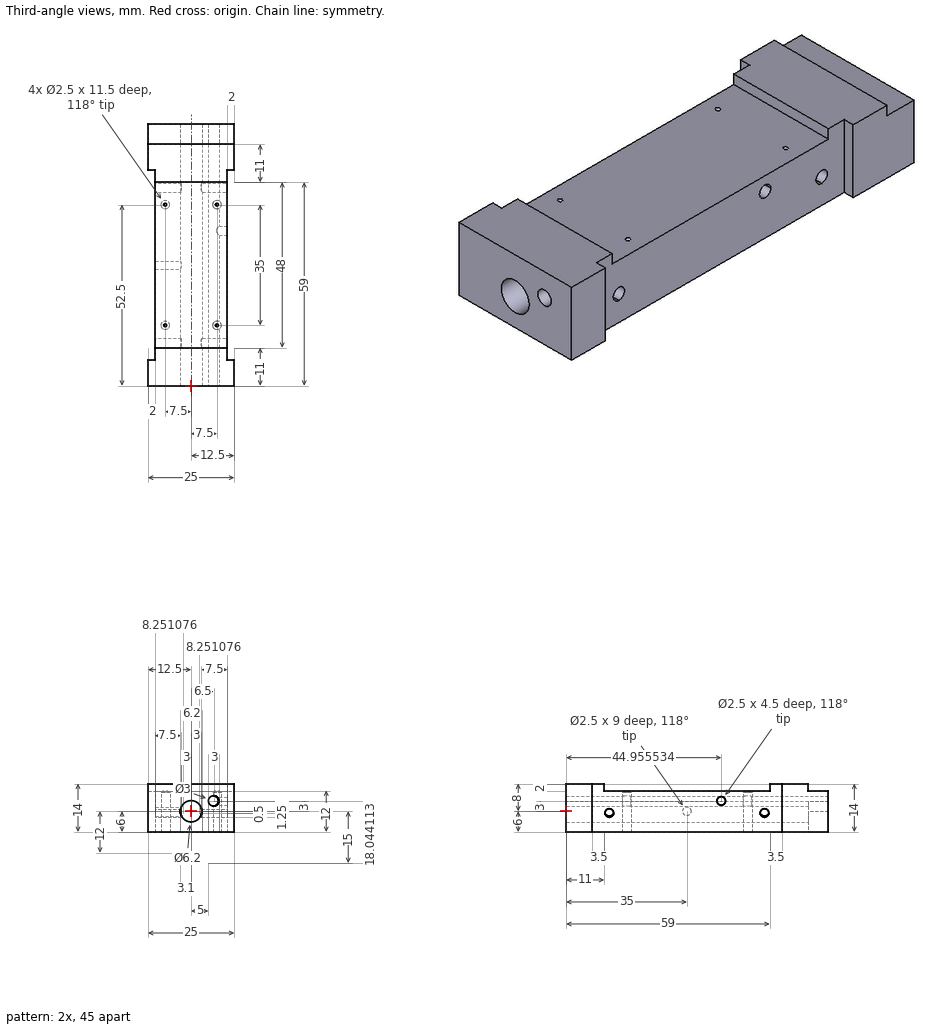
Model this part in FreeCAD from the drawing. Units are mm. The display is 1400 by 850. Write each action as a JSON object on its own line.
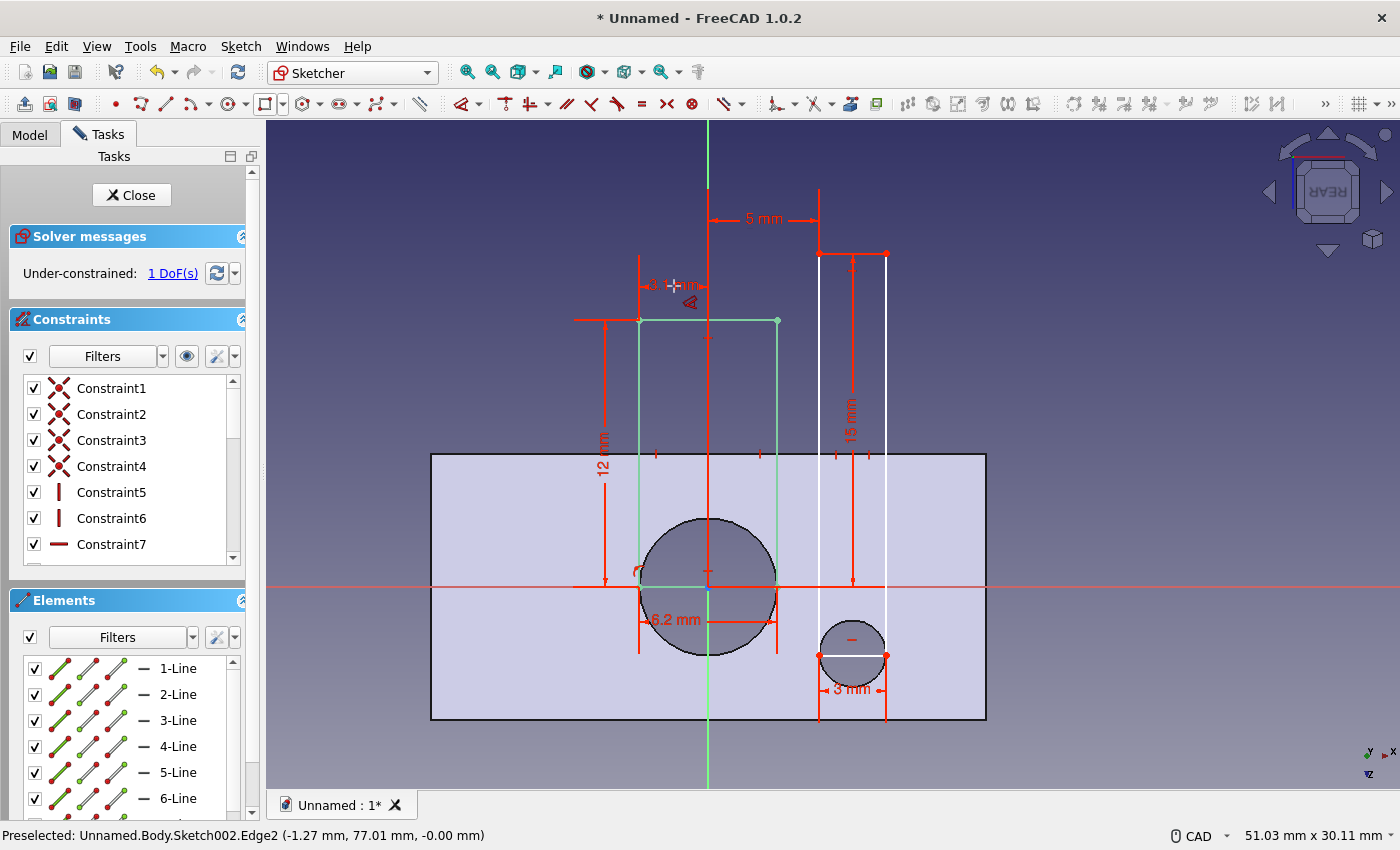
{"action": "left_click", "coordinate": [819, 374]}
{"action": "left_click", "coordinate": [853, 455]}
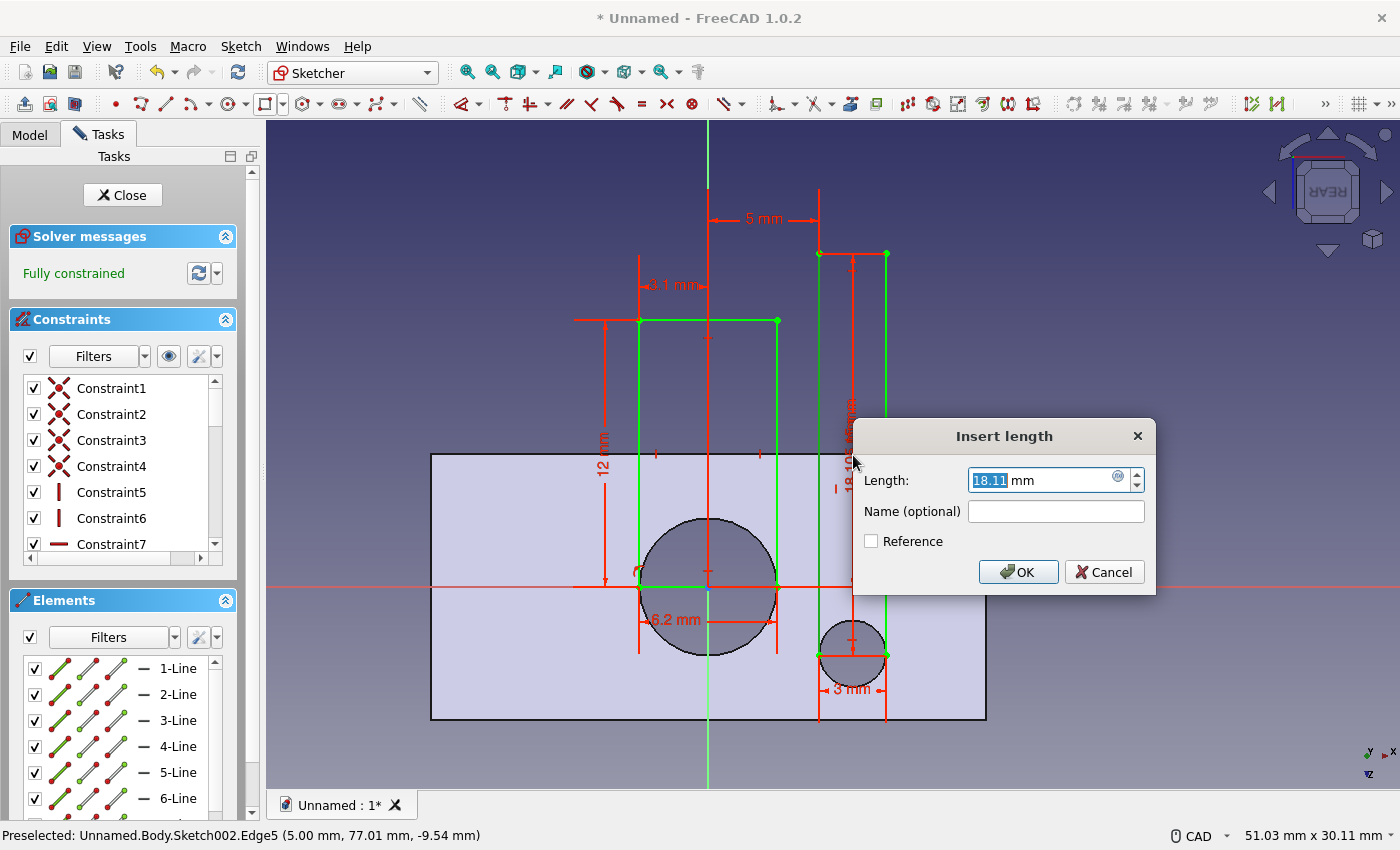
{"action": "type", "text": "18.044113"}
{"action": "key", "text": "Return"}
{"action": "key", "text": "Escape"}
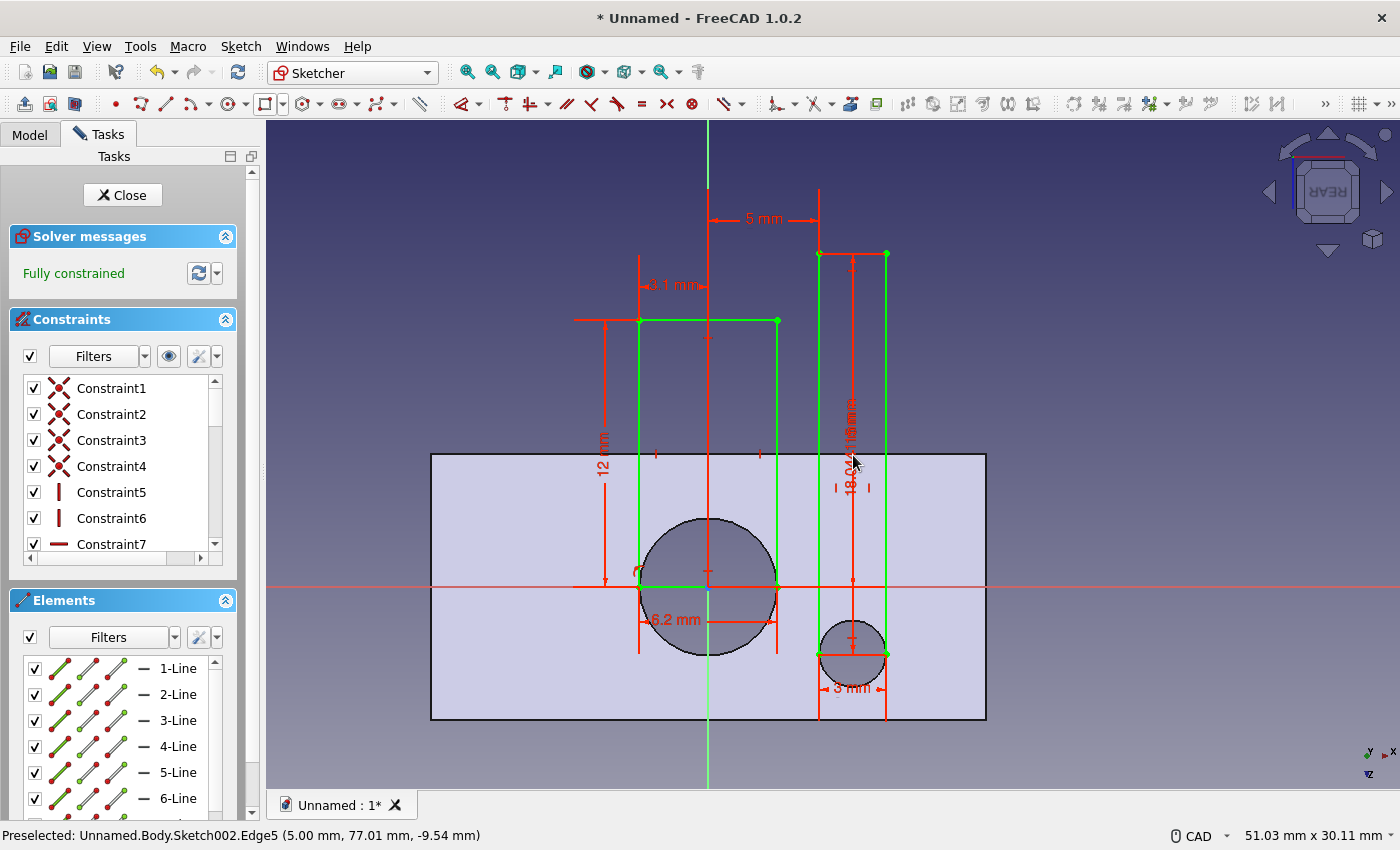
{"action": "left_click", "coordinate": [123, 195]}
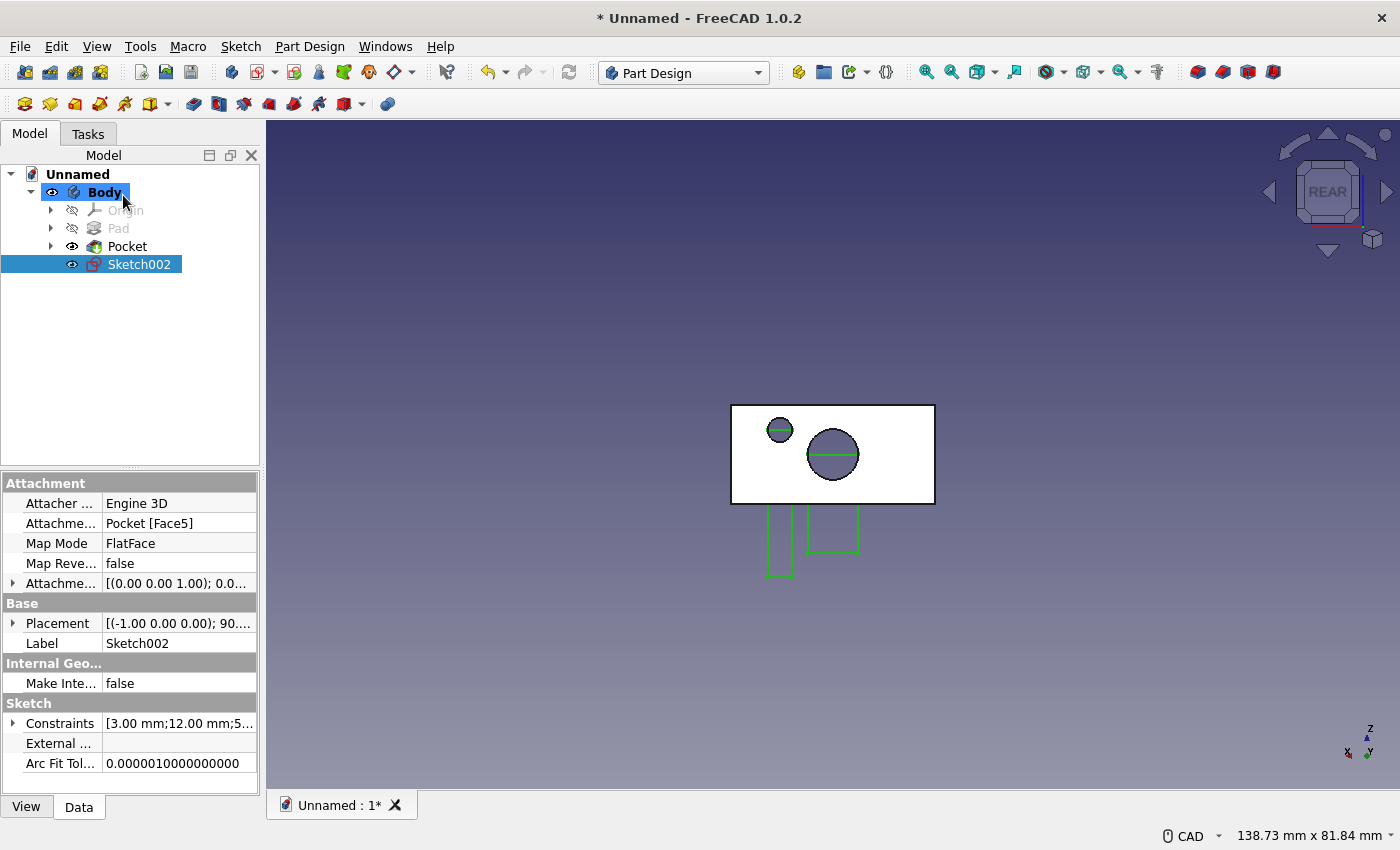
{"action": "left_click", "coordinate": [194, 104]}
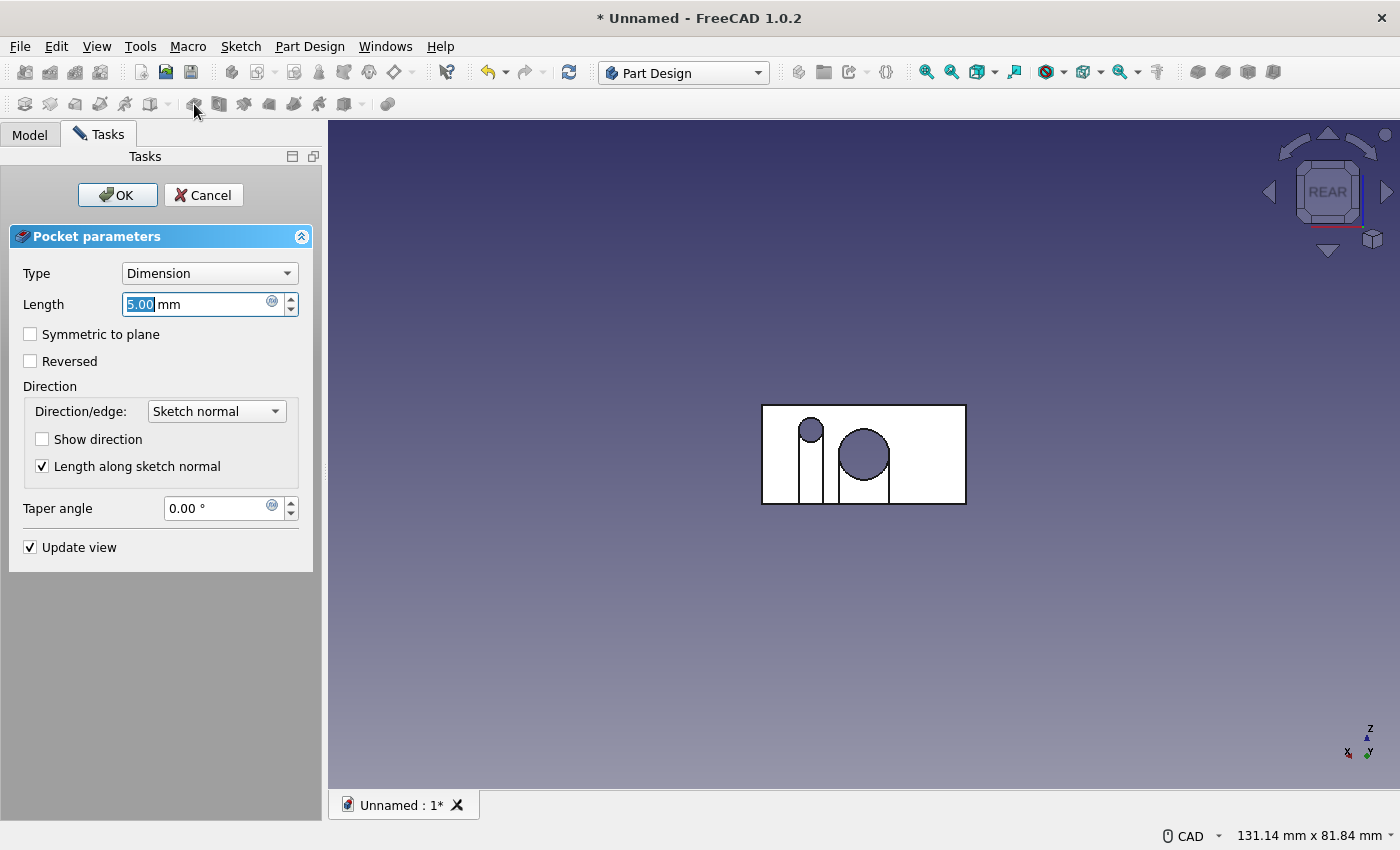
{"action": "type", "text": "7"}
{"action": "key", "text": "Tab"}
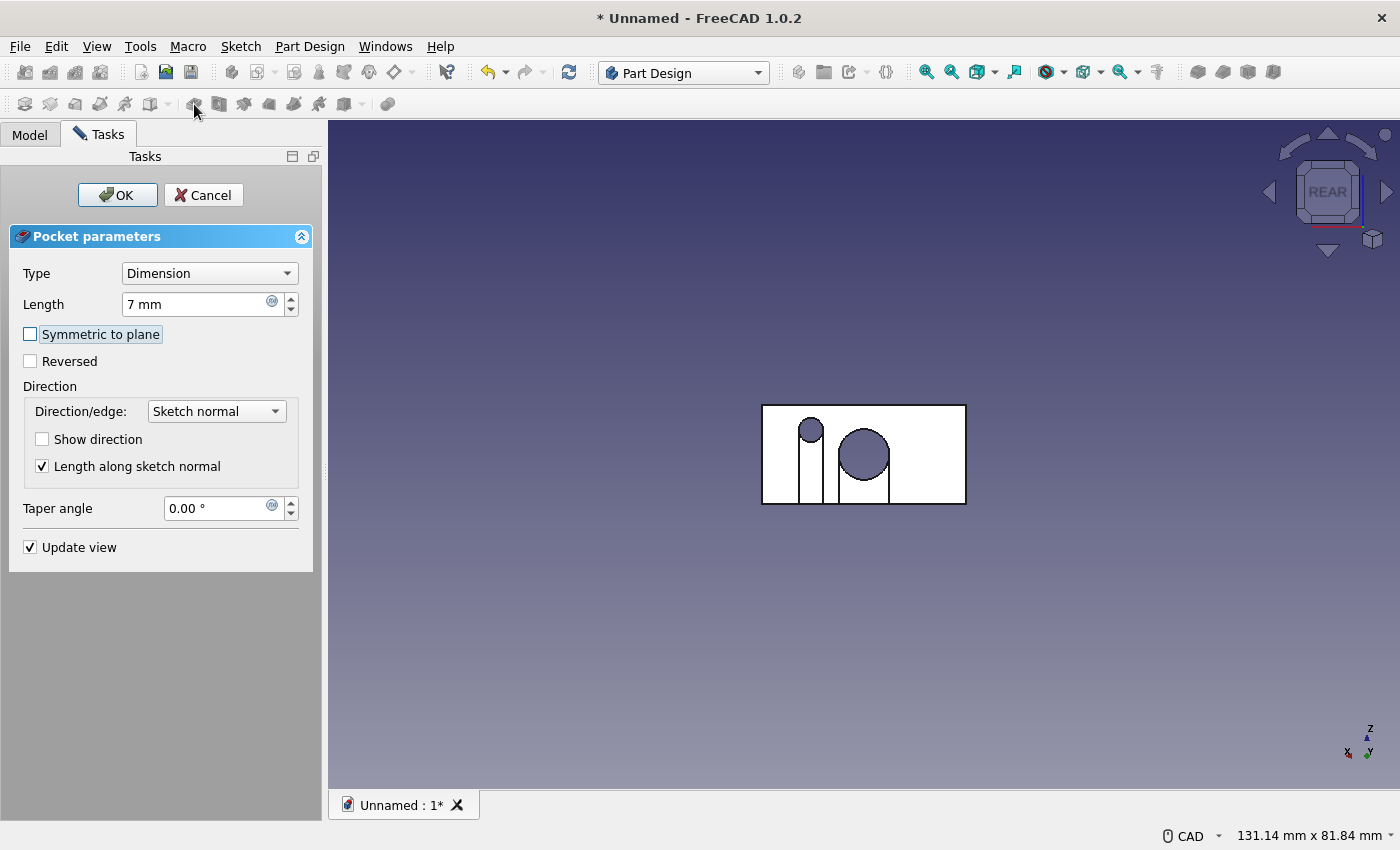
{"action": "left_click", "coordinate": [118, 195]}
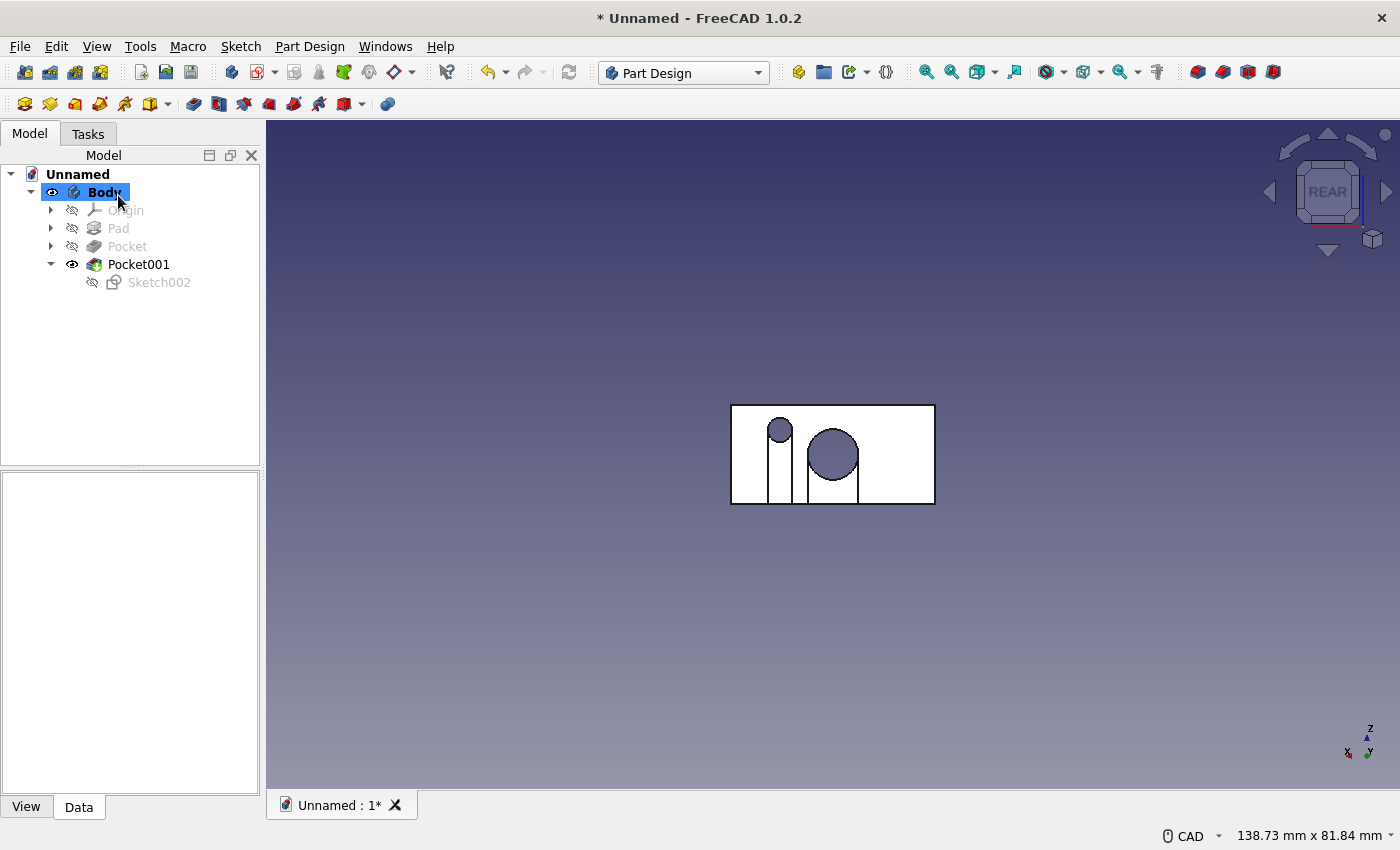
{"action": "left_click", "coordinate": [927, 72]}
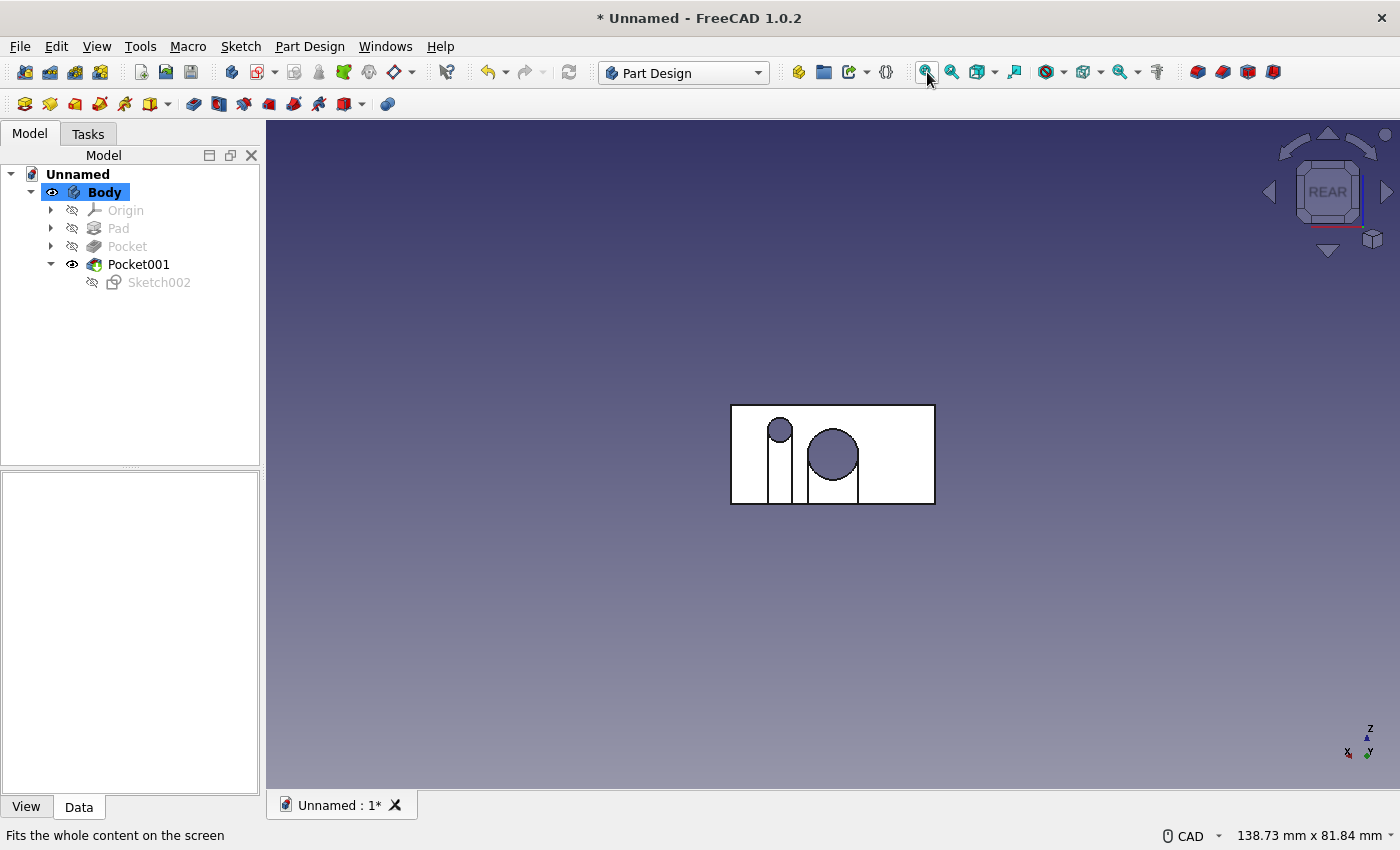
{"action": "key", "text": "0"}